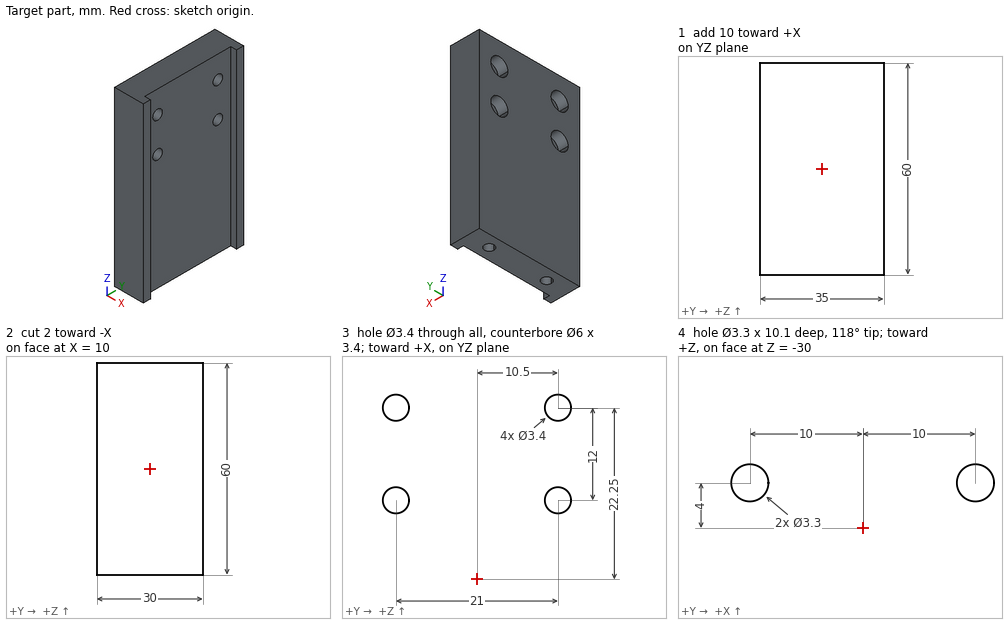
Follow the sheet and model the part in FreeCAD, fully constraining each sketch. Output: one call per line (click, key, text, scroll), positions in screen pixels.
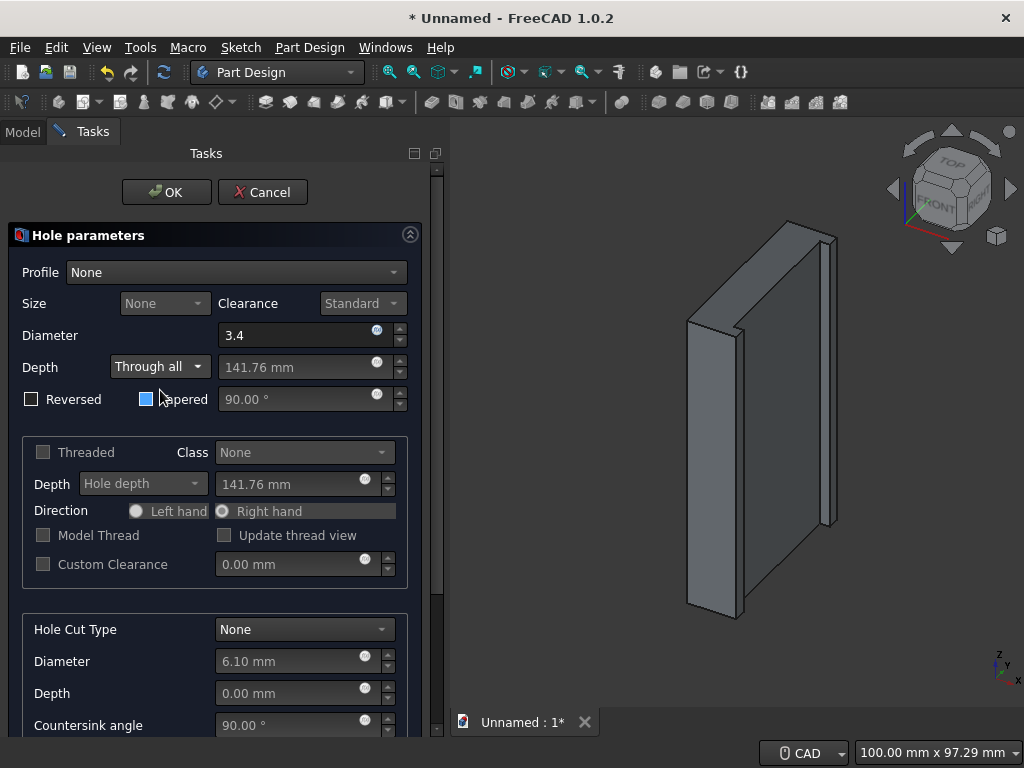
click(30, 399)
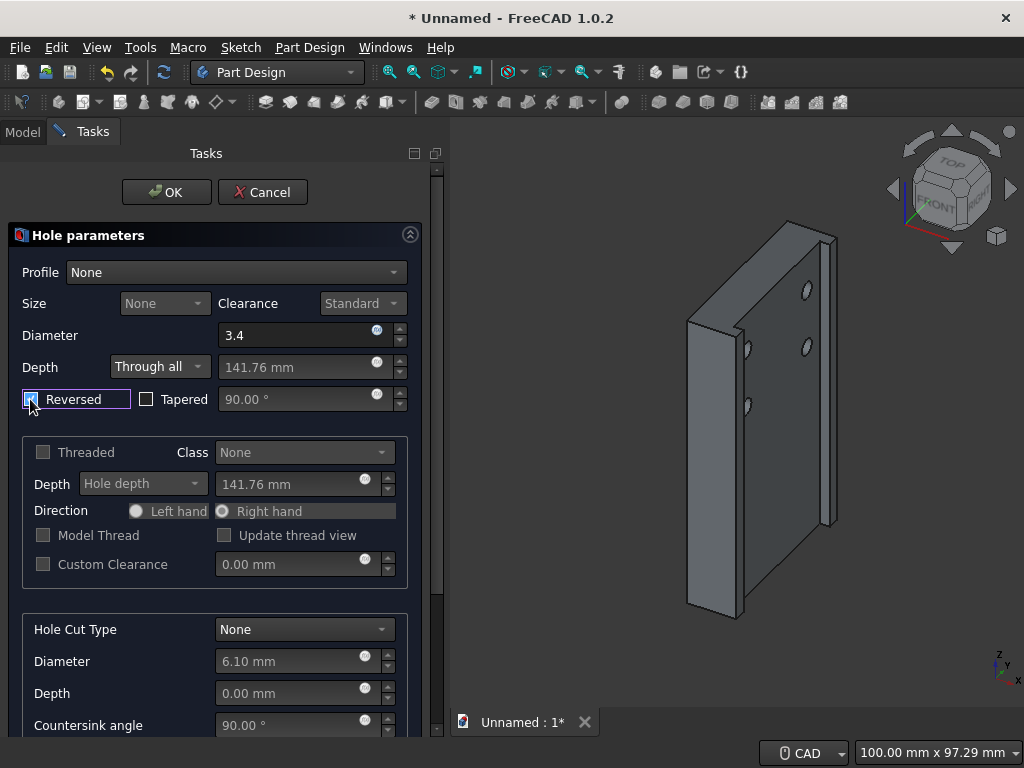
click(306, 630)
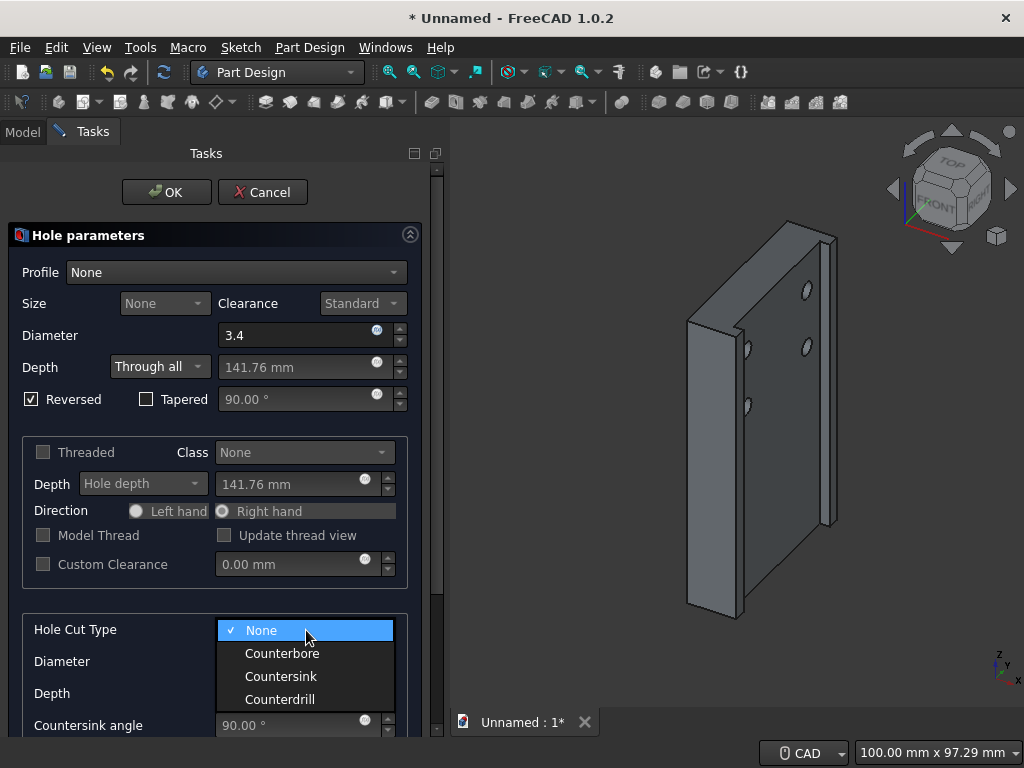
click(304, 654)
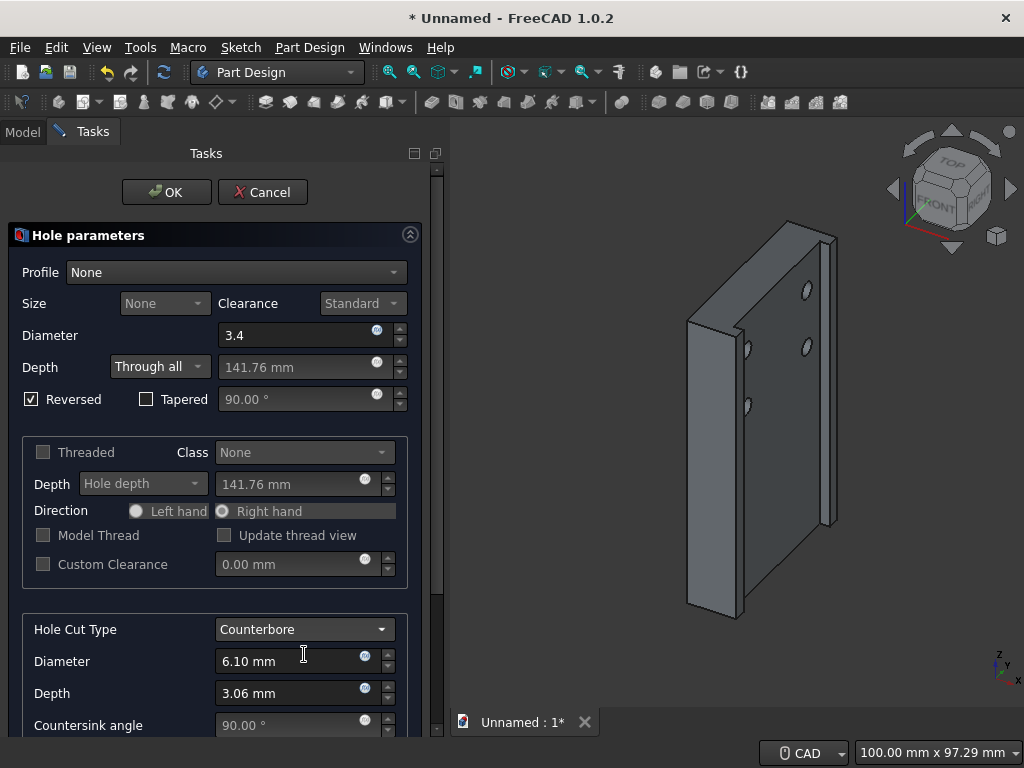
triple_click(298, 661)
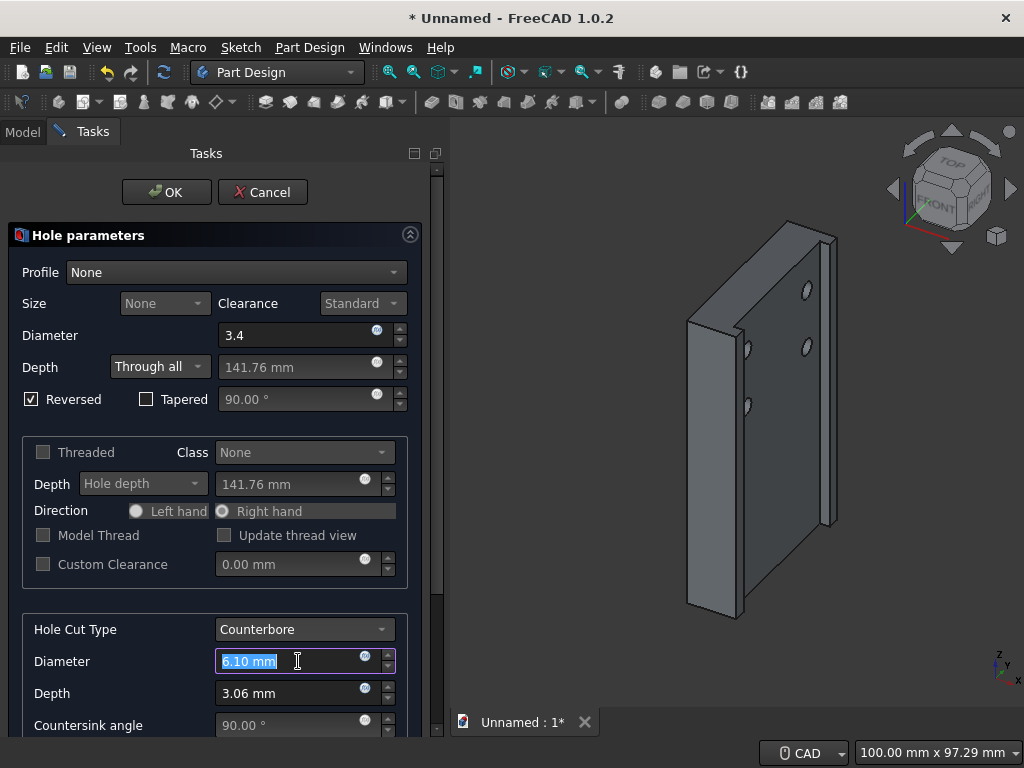
text(6)
key(Tab)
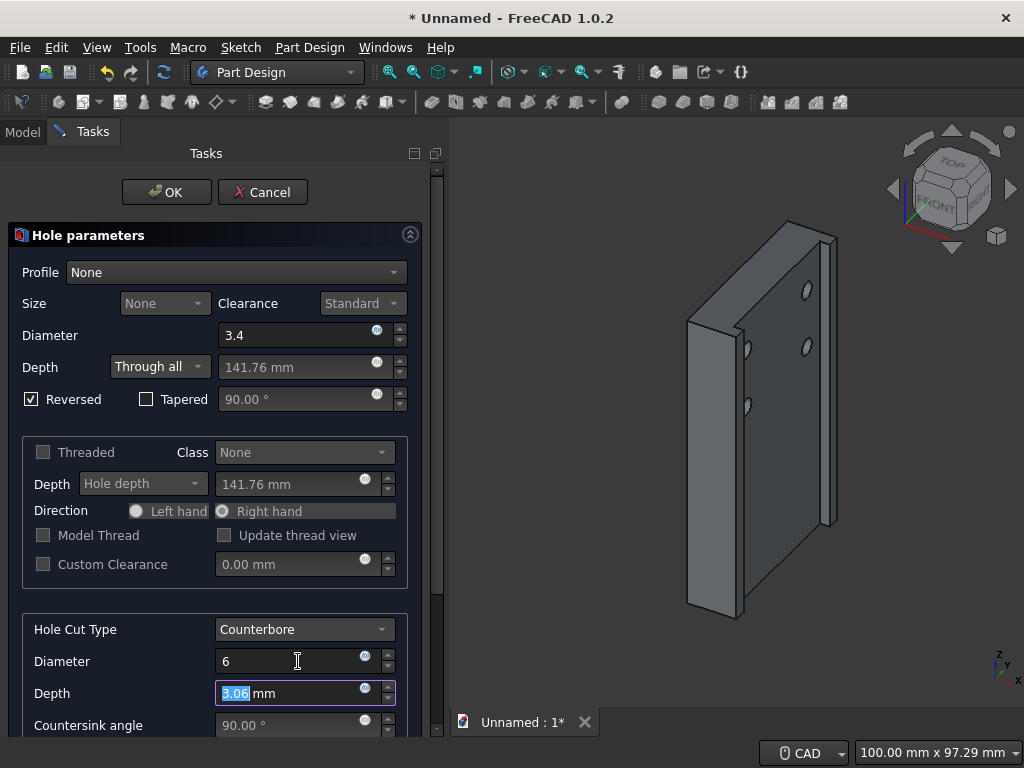
text(3.4)
key(Tab)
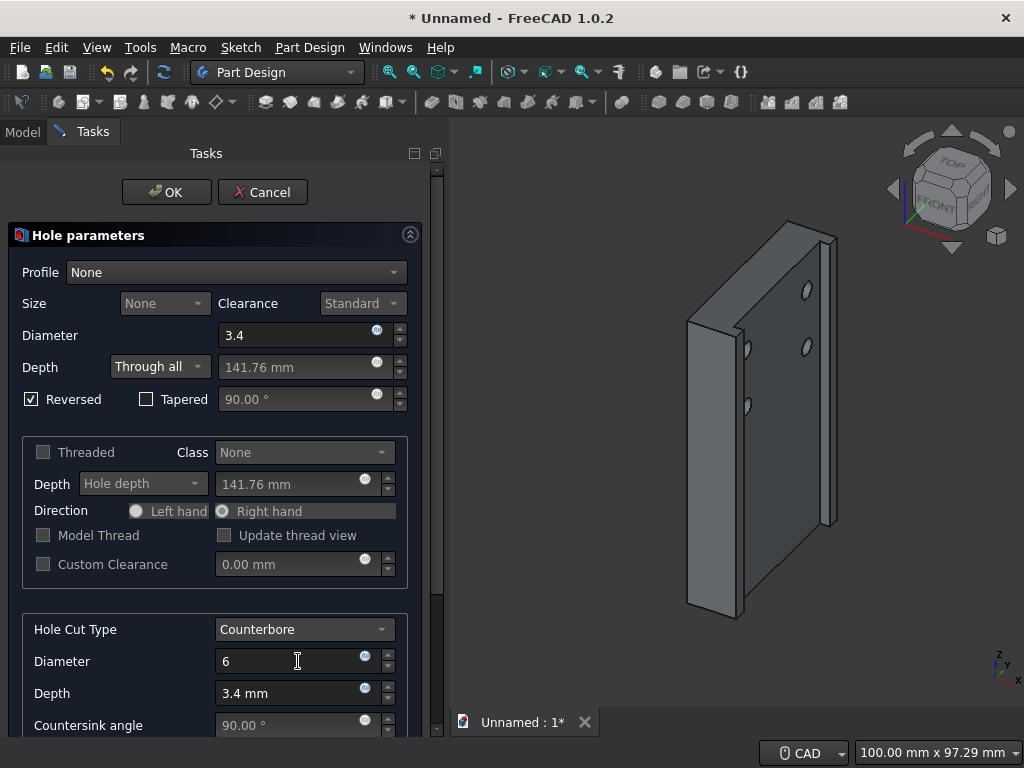
click(167, 192)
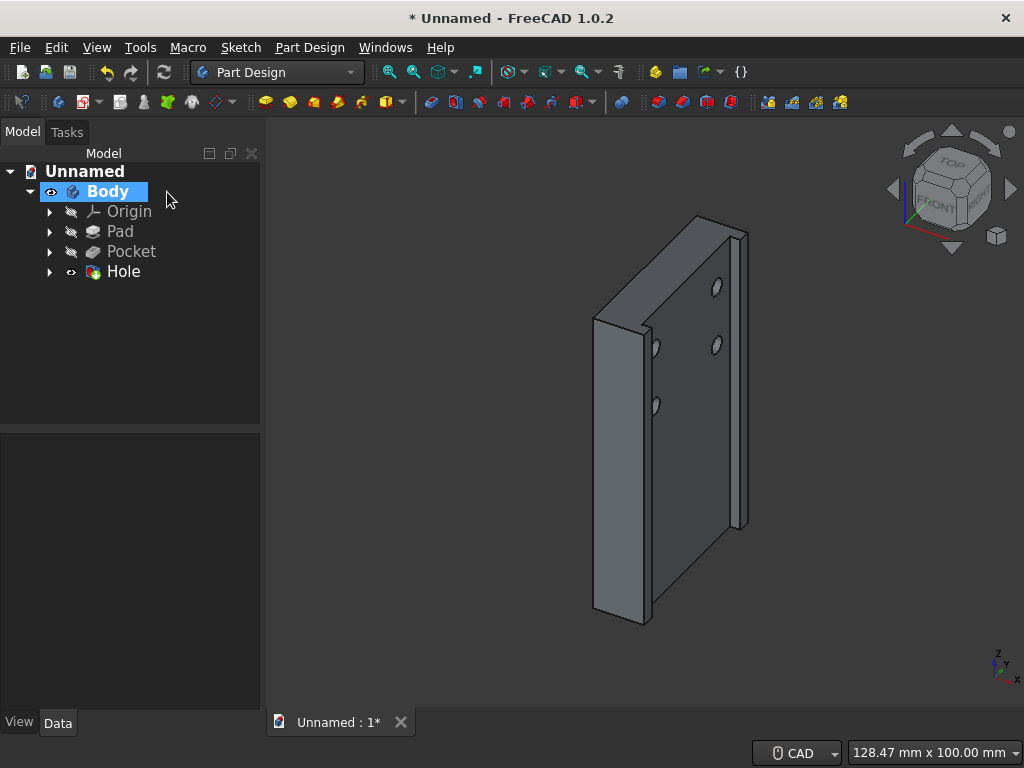
key(5)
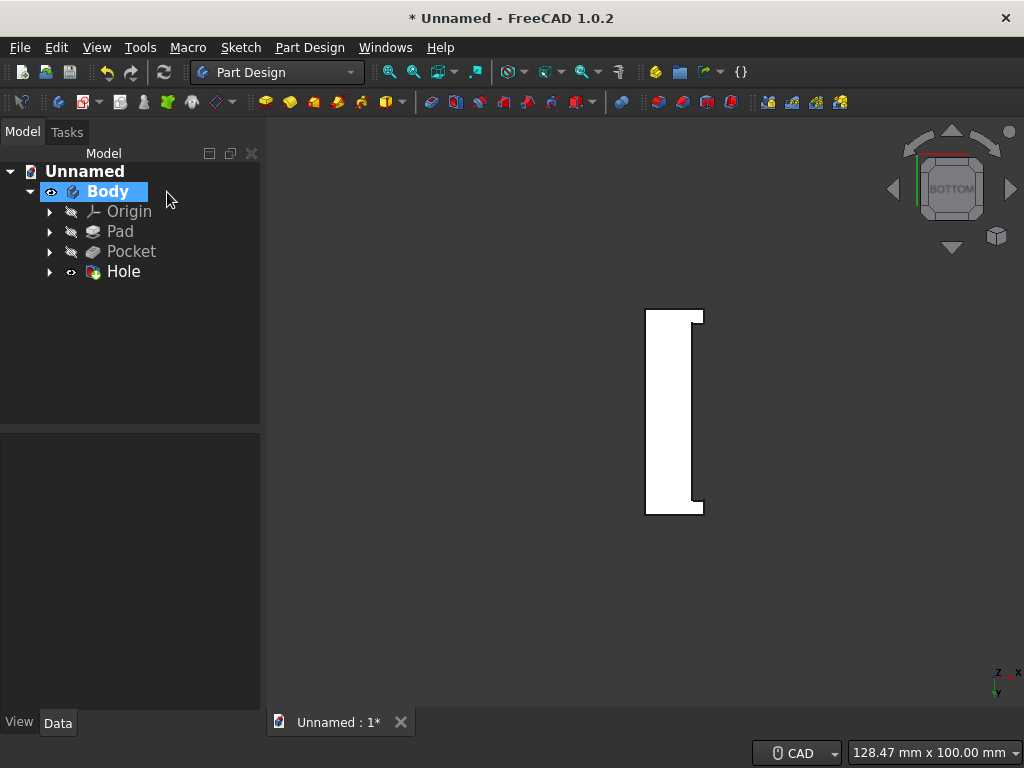
key(v)
key(f)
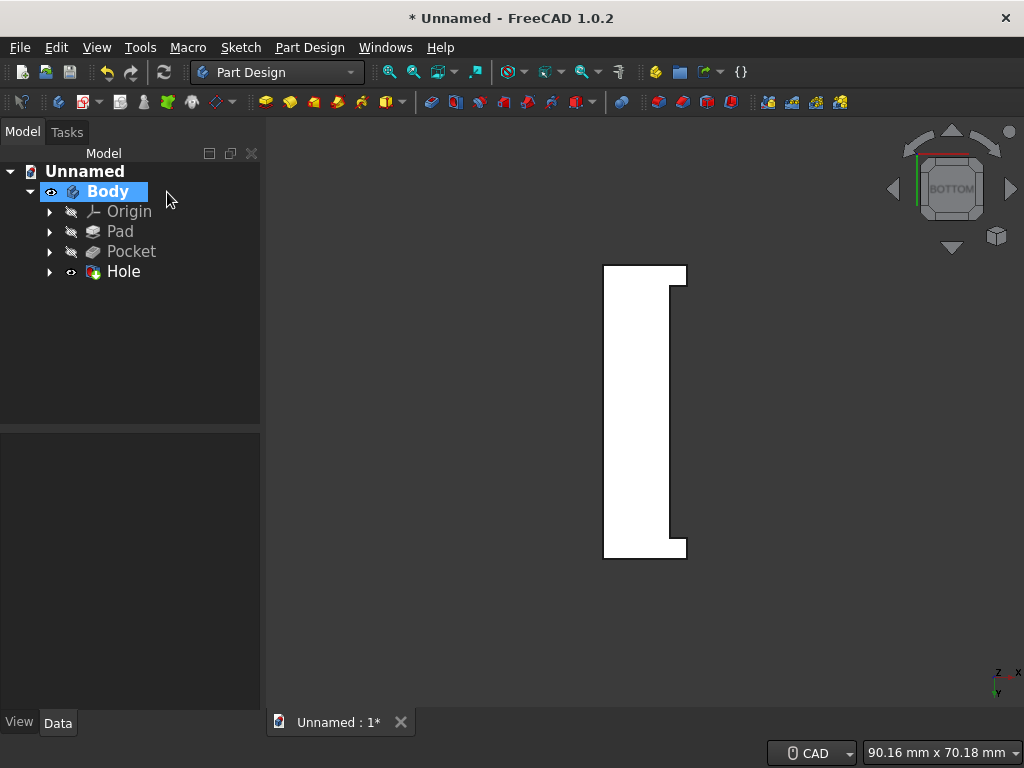
click(633, 495)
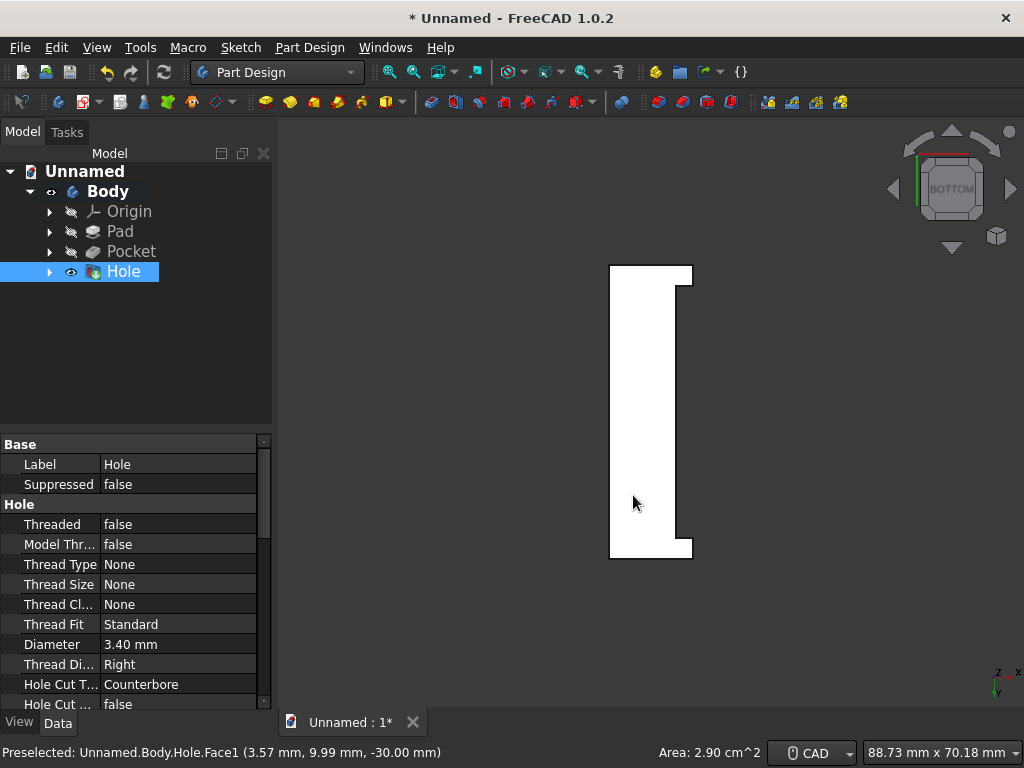
click(84, 102)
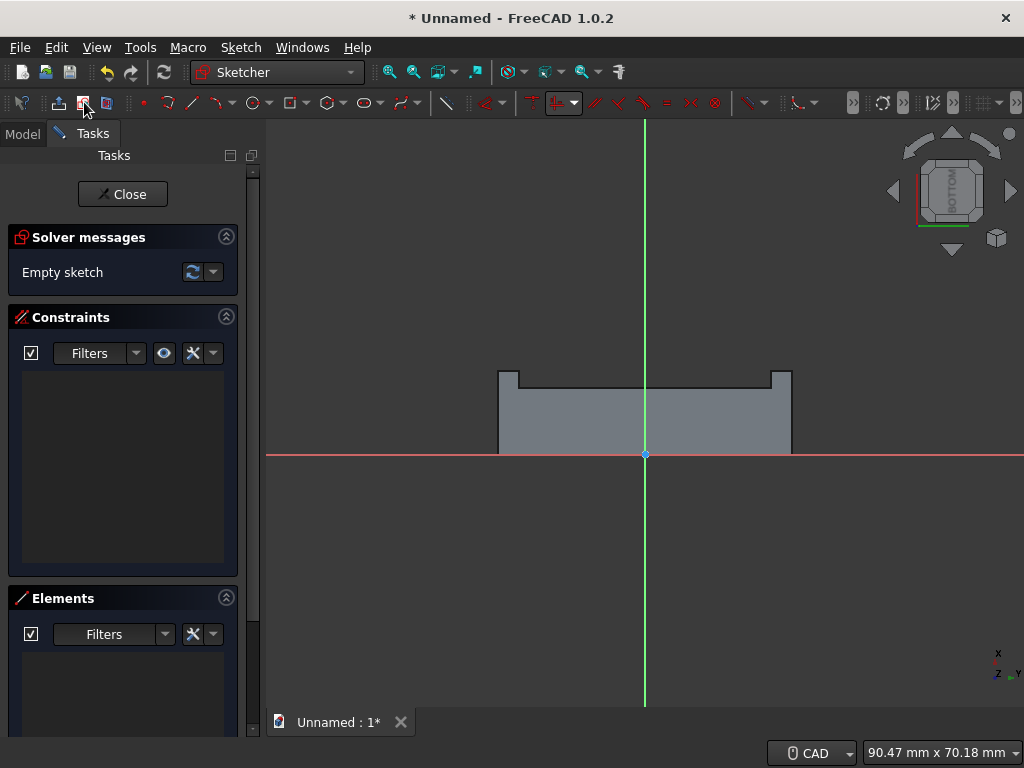
scroll(701, 446, up, 4)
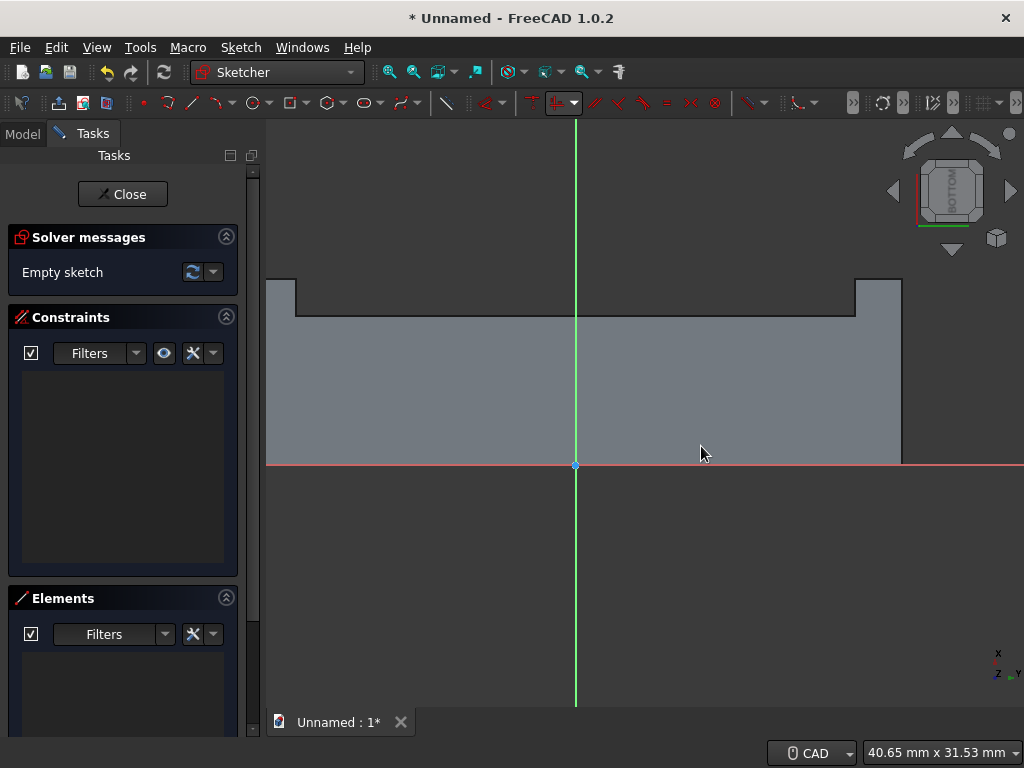
key(g)
key(c)